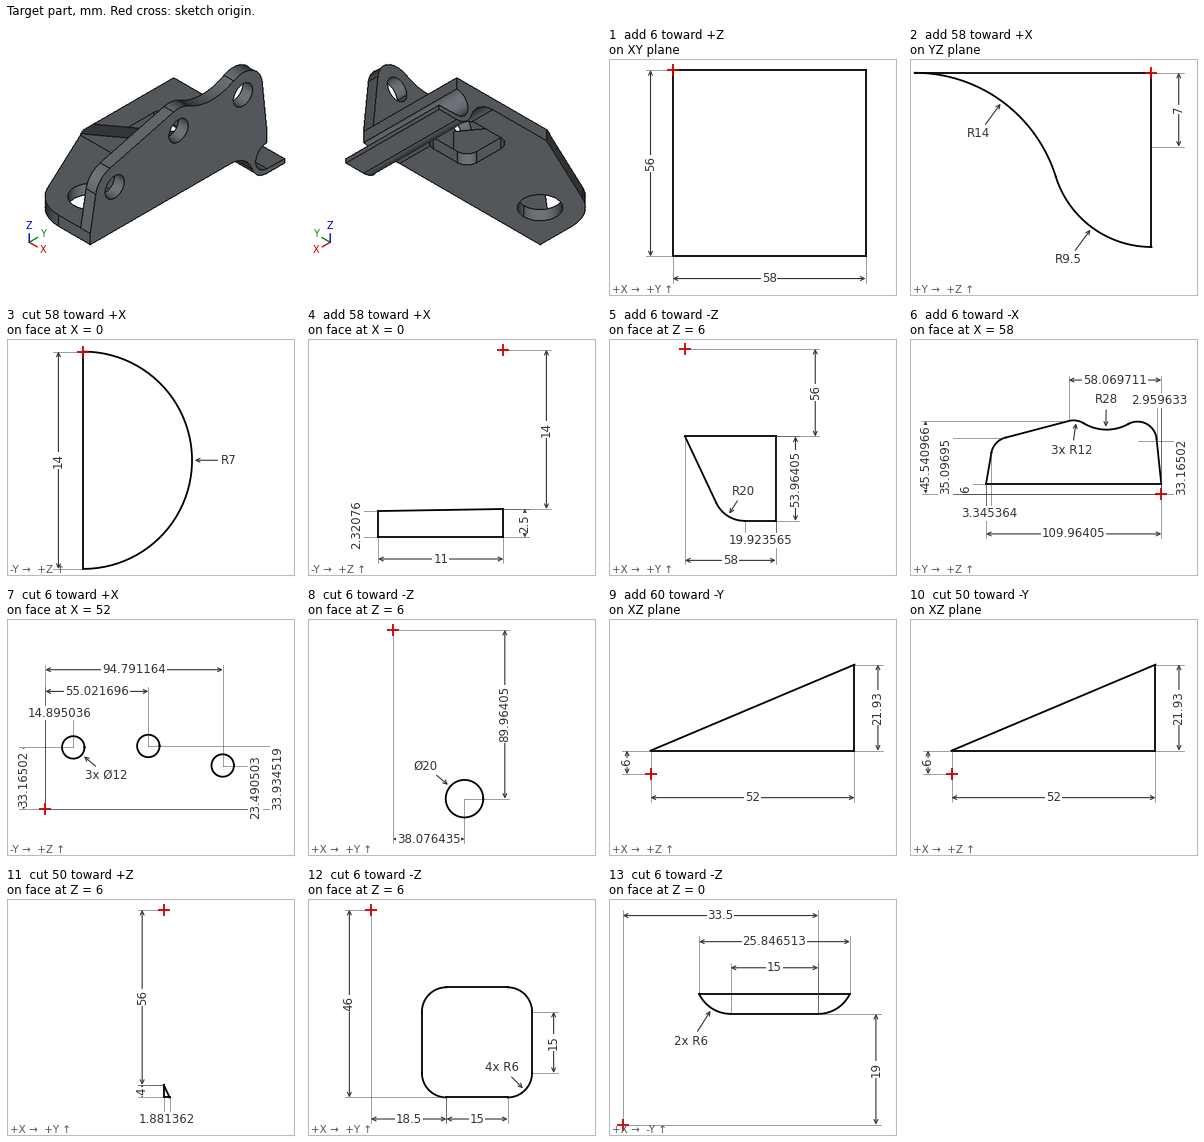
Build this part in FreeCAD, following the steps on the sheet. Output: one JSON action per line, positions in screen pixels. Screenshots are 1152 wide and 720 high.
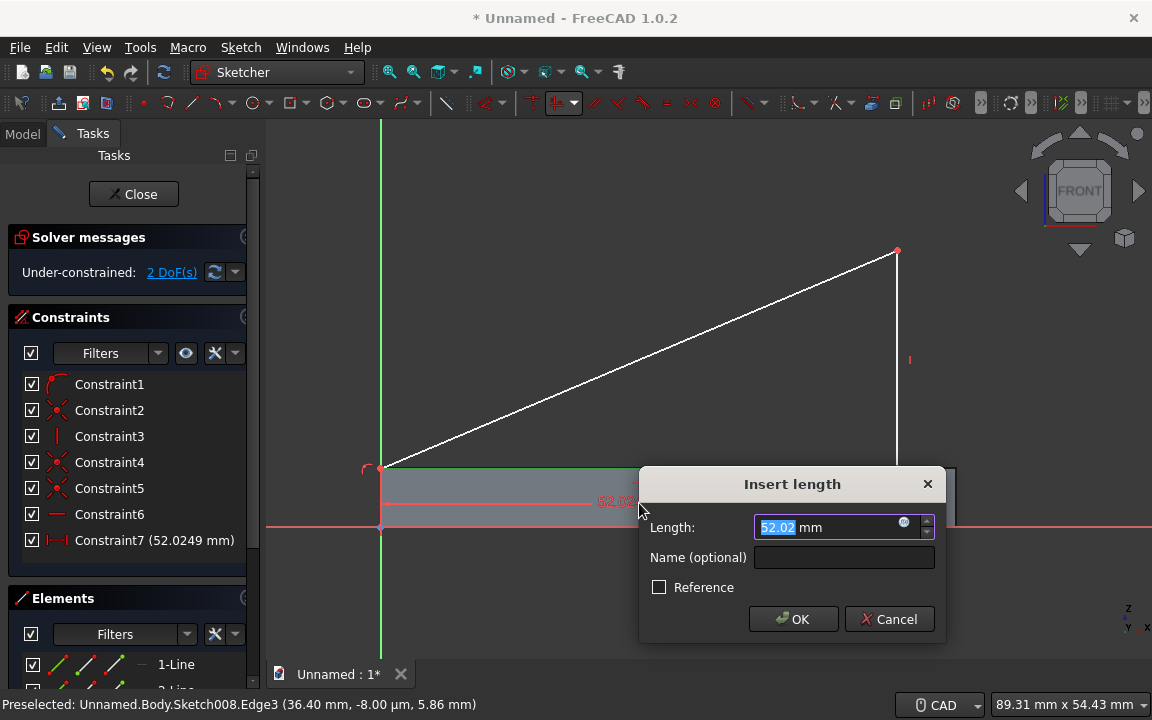
{"action": "type", "text": "52"}
{"action": "key", "text": "Return"}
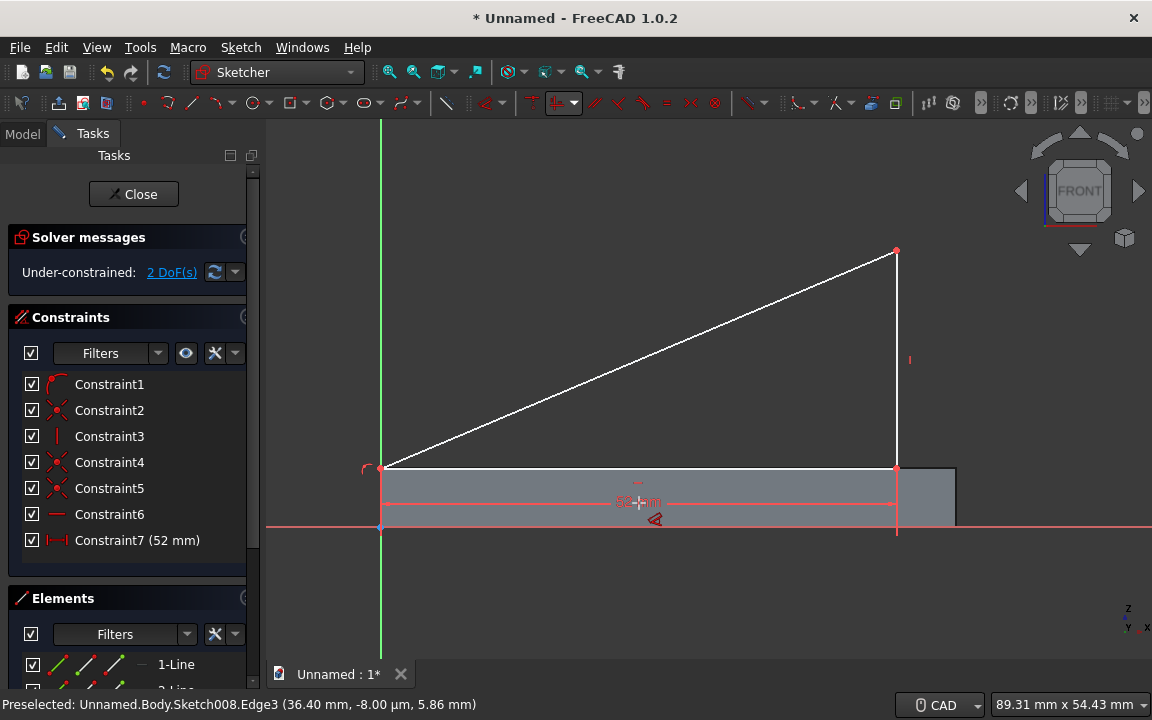
{"action": "left_click", "coordinate": [381, 469]}
{"action": "left_click", "coordinate": [347, 498]}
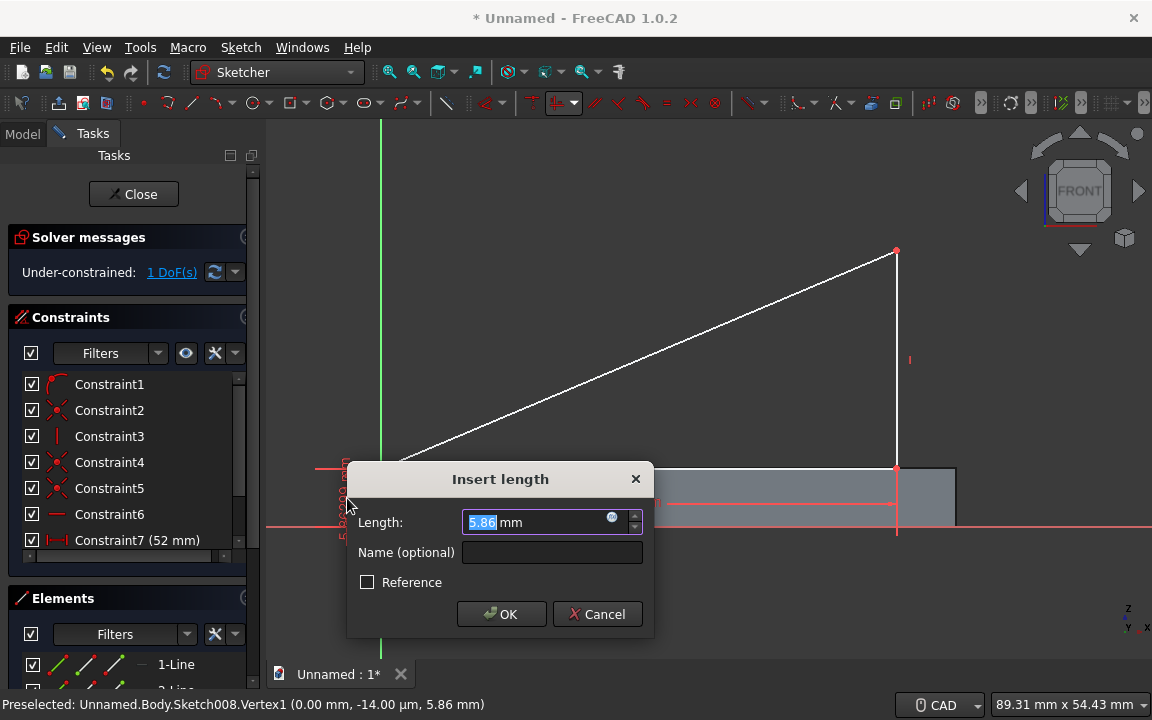
{"action": "type", "text": "6"}
{"action": "key", "text": "Return"}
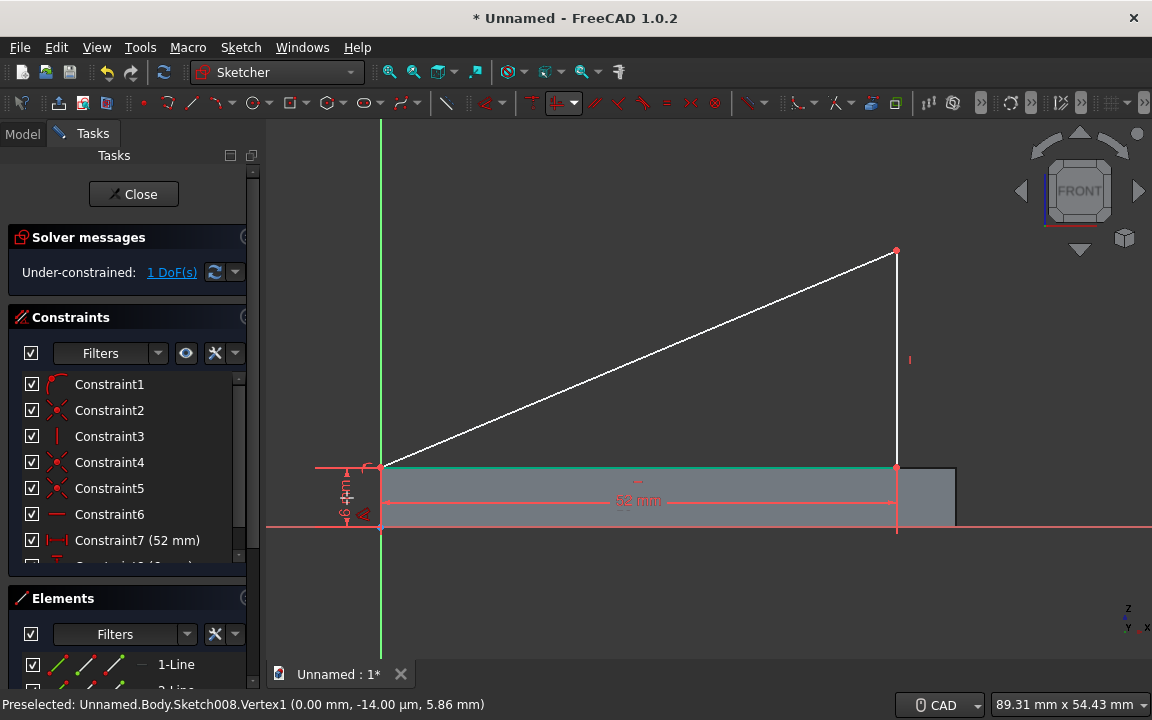
{"action": "left_click", "coordinate": [897, 316]}
{"action": "left_click", "coordinate": [931, 359]}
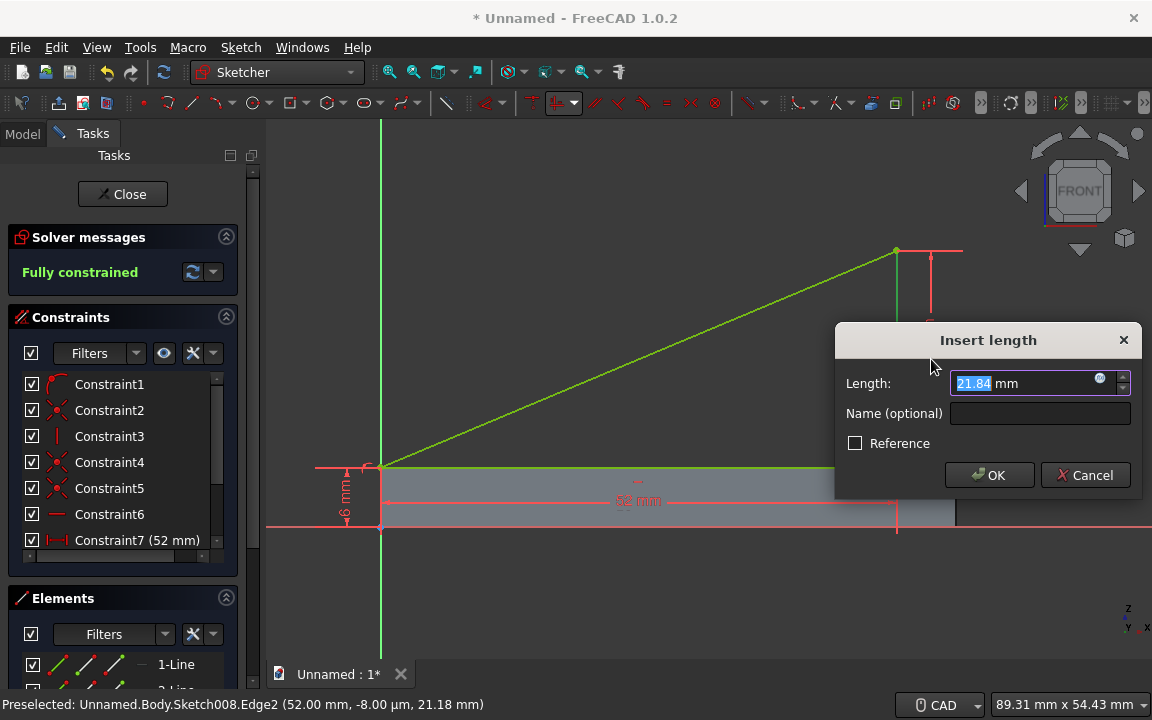
{"action": "type", "text": "21.93"}
{"action": "key", "text": "Return"}
{"action": "key", "text": "Escape"}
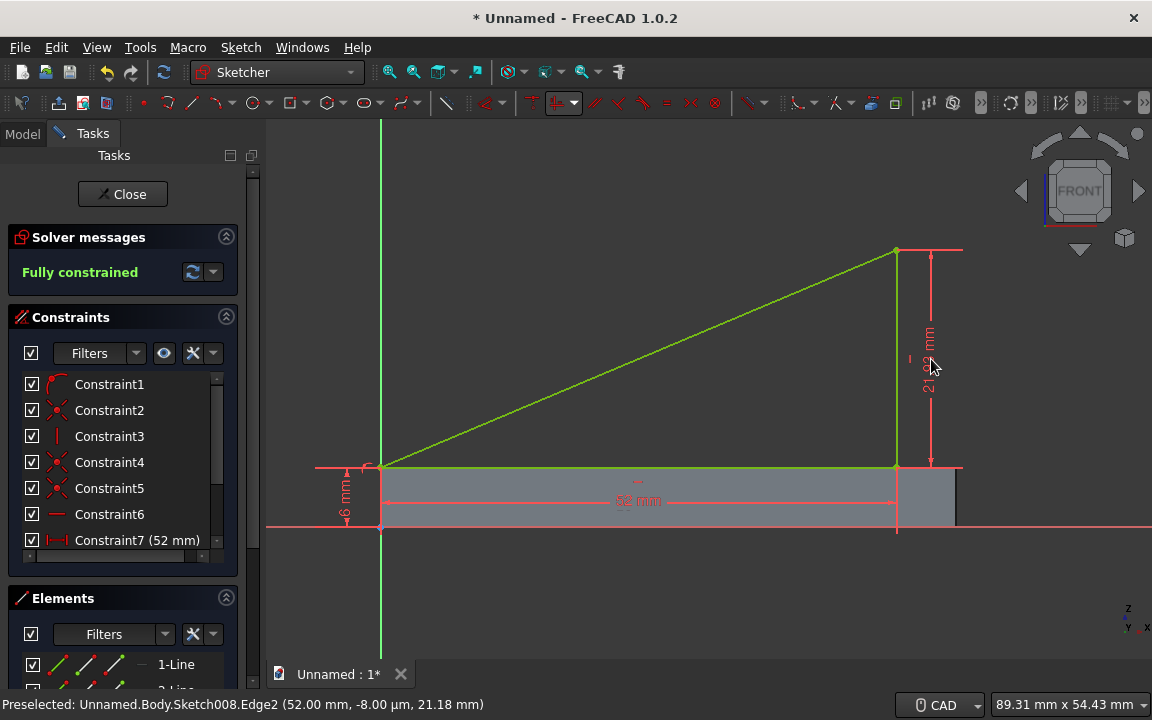
{"action": "left_click", "coordinate": [123, 194]}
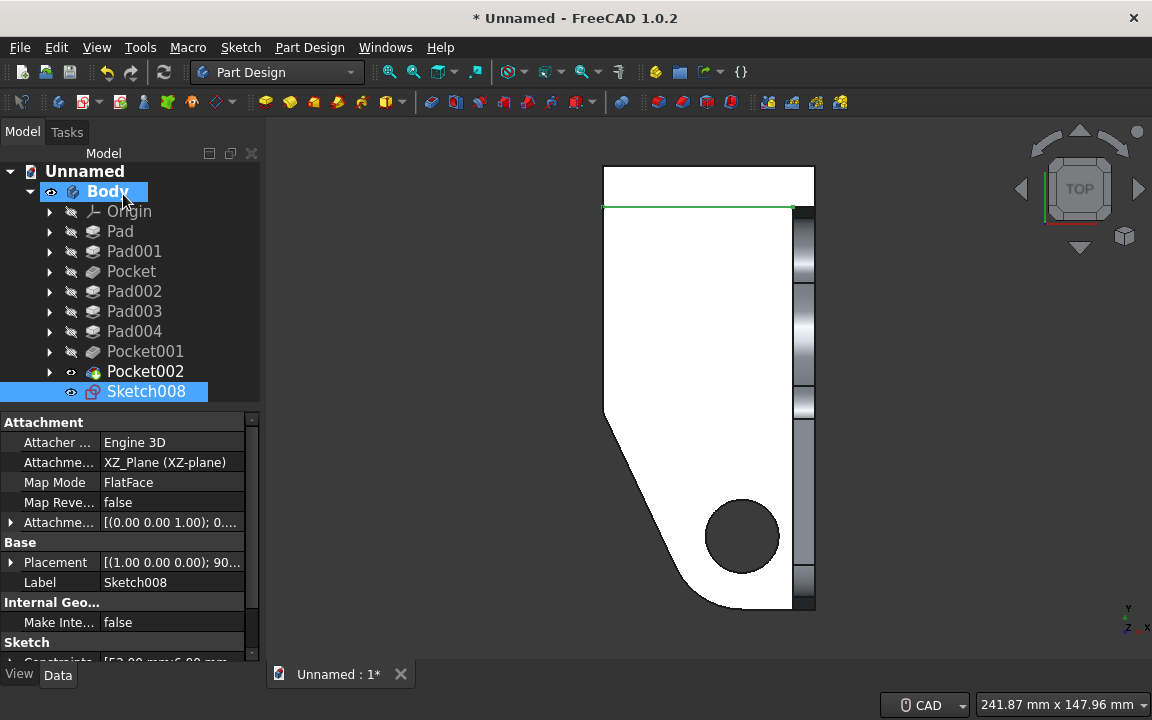
{"action": "left_click", "coordinate": [266, 102]}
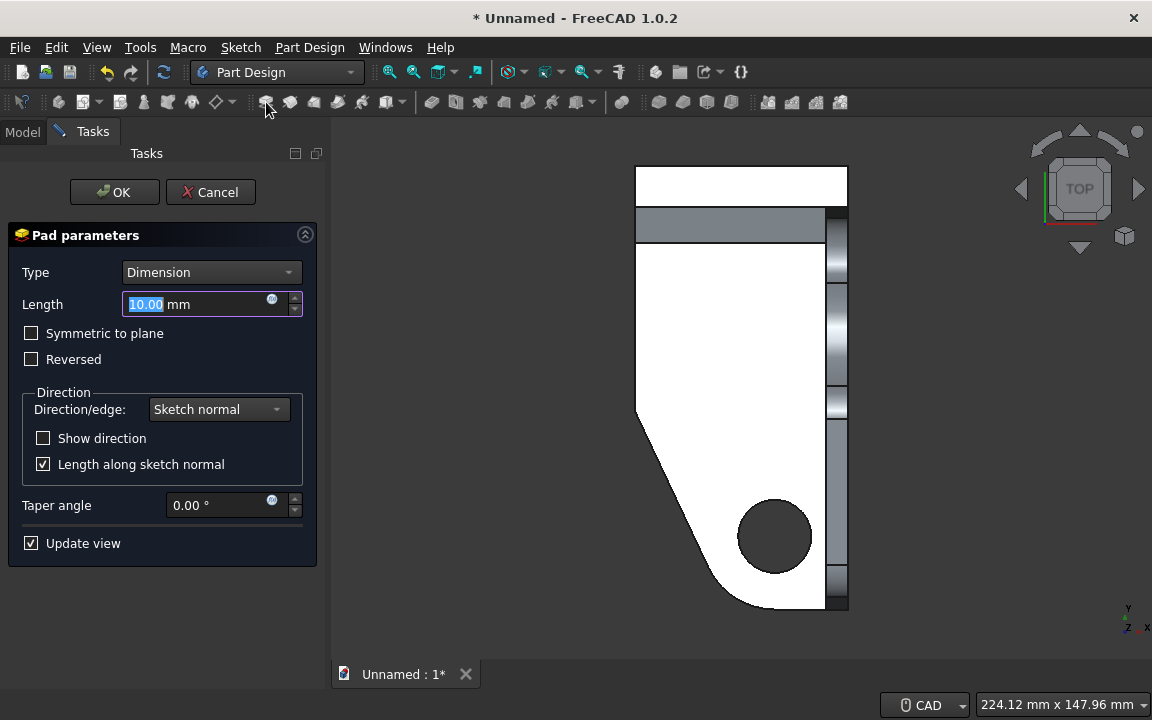
{"action": "type", "text": "60"}
{"action": "key", "text": "Tab"}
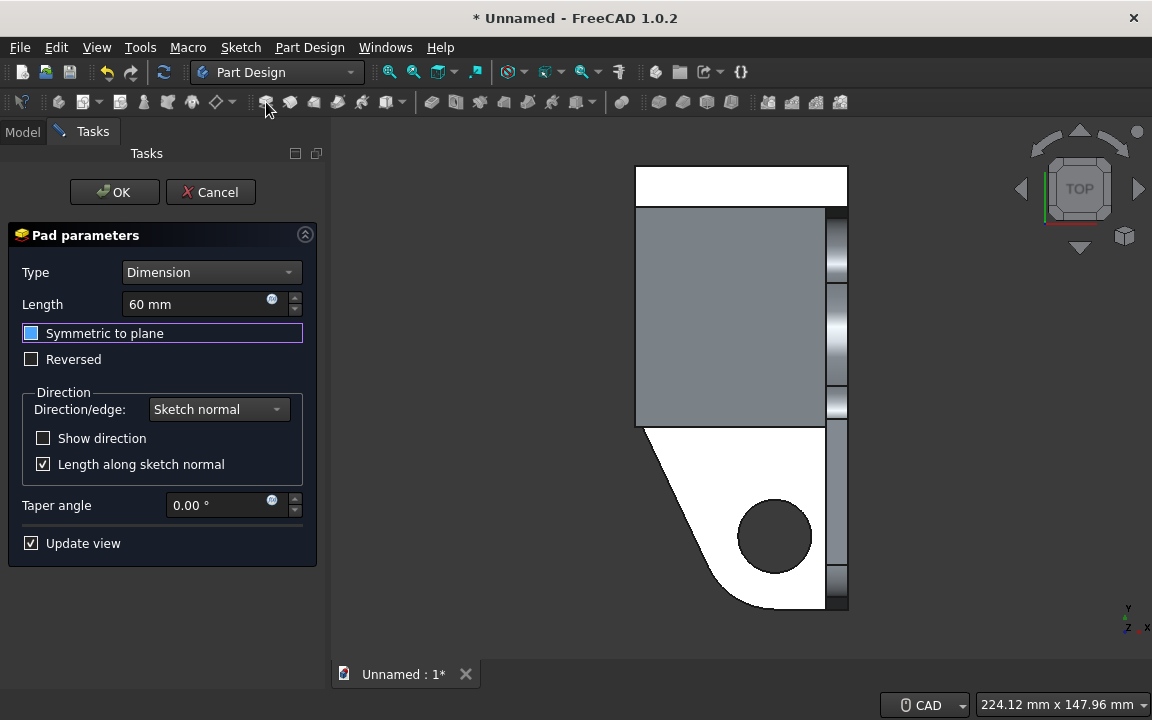
{"action": "left_click", "coordinate": [115, 192]}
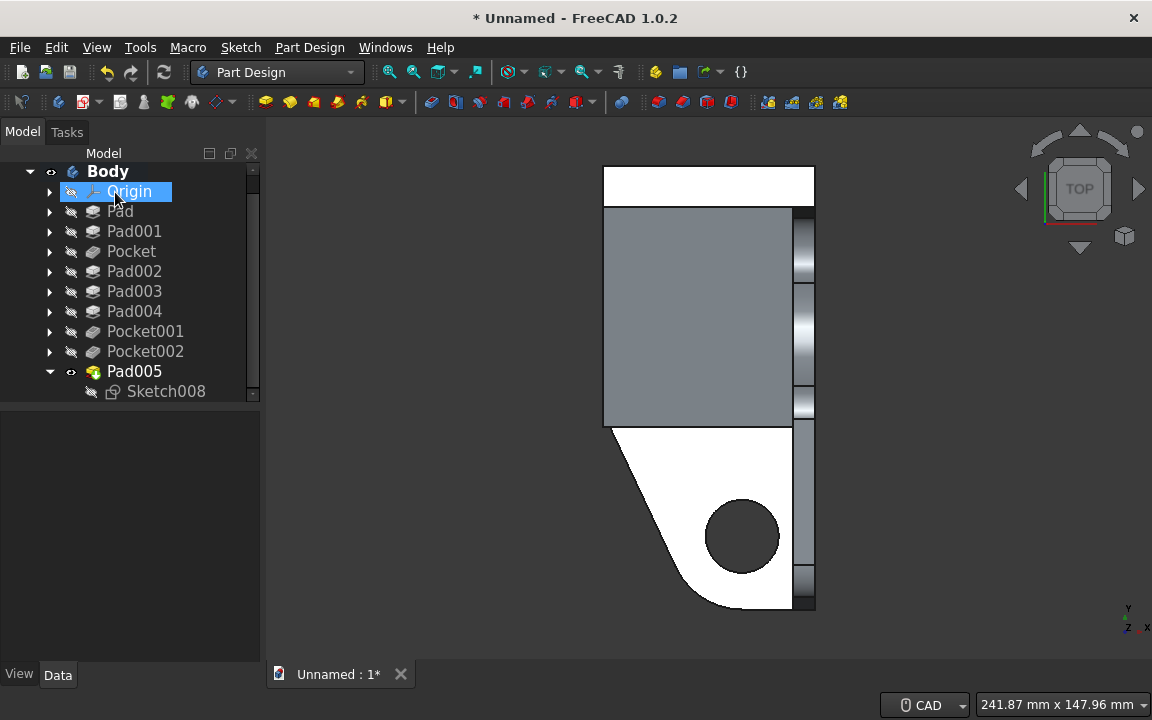
{"action": "left_click", "coordinate": [84, 102]}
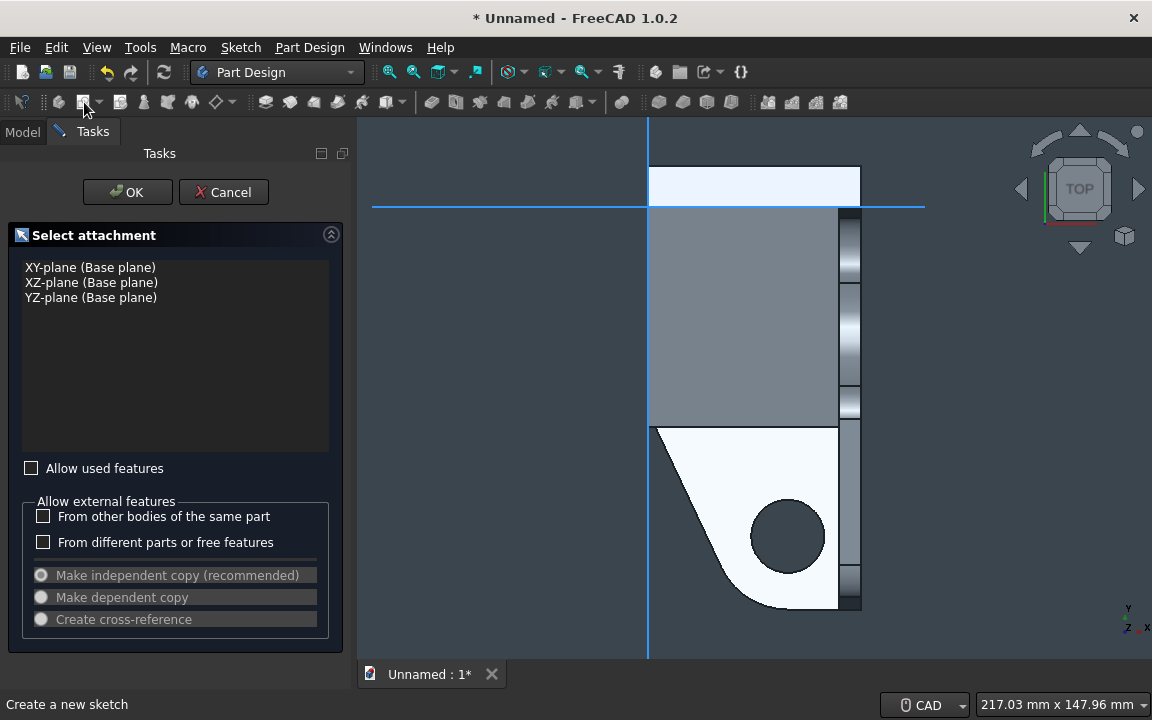
{"action": "left_click", "coordinate": [82, 282]}